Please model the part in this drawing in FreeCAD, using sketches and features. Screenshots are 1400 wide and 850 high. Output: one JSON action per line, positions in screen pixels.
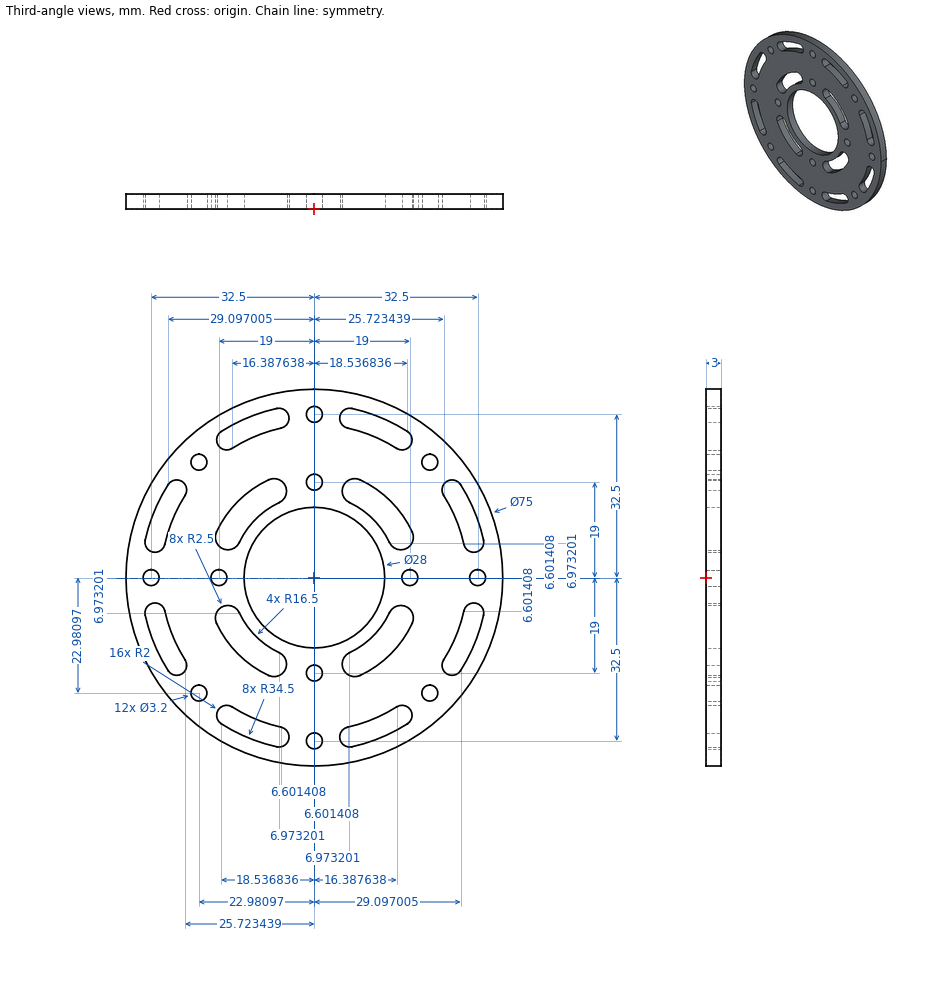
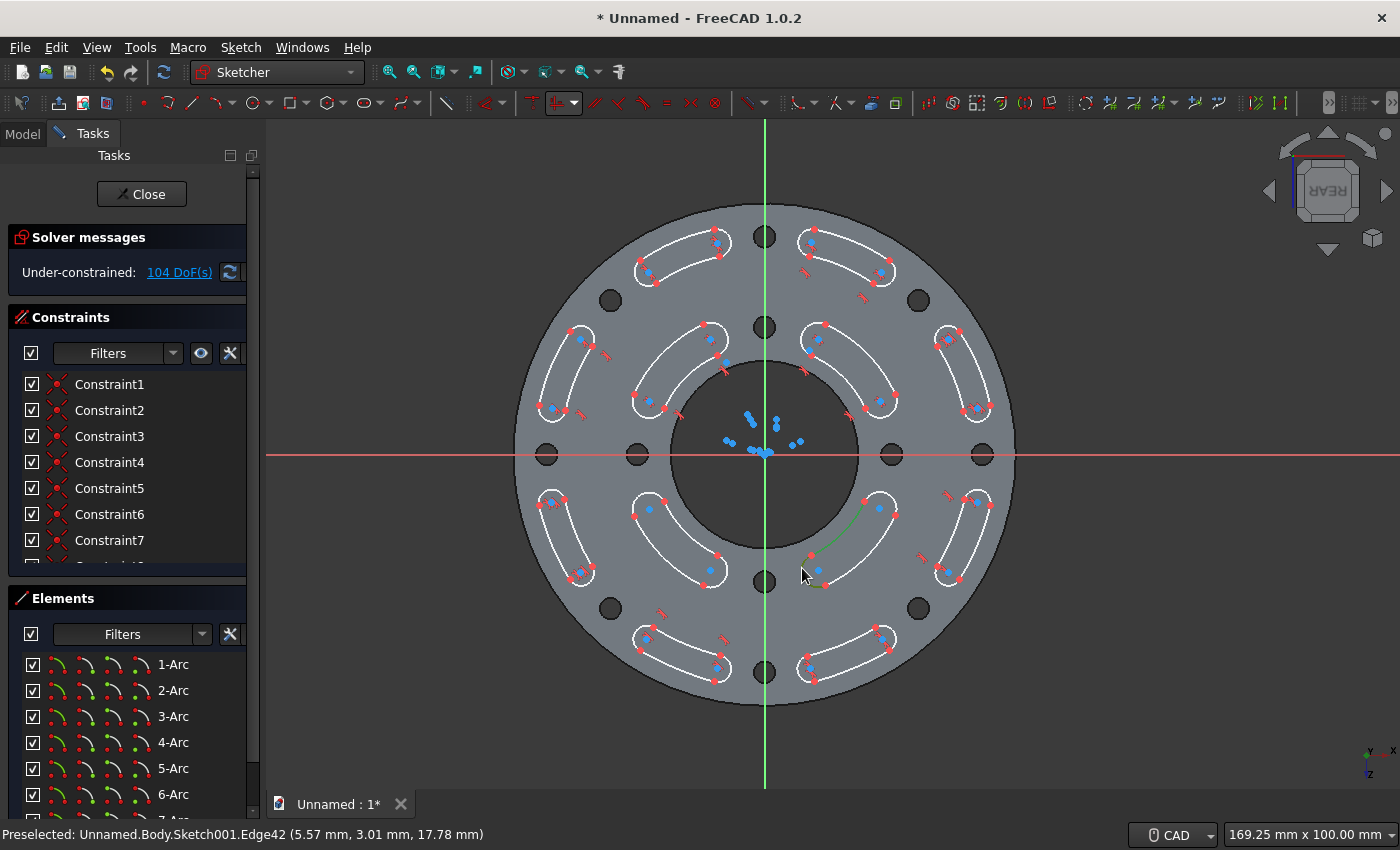
{"action": "left_click", "coordinate": [644, 104]}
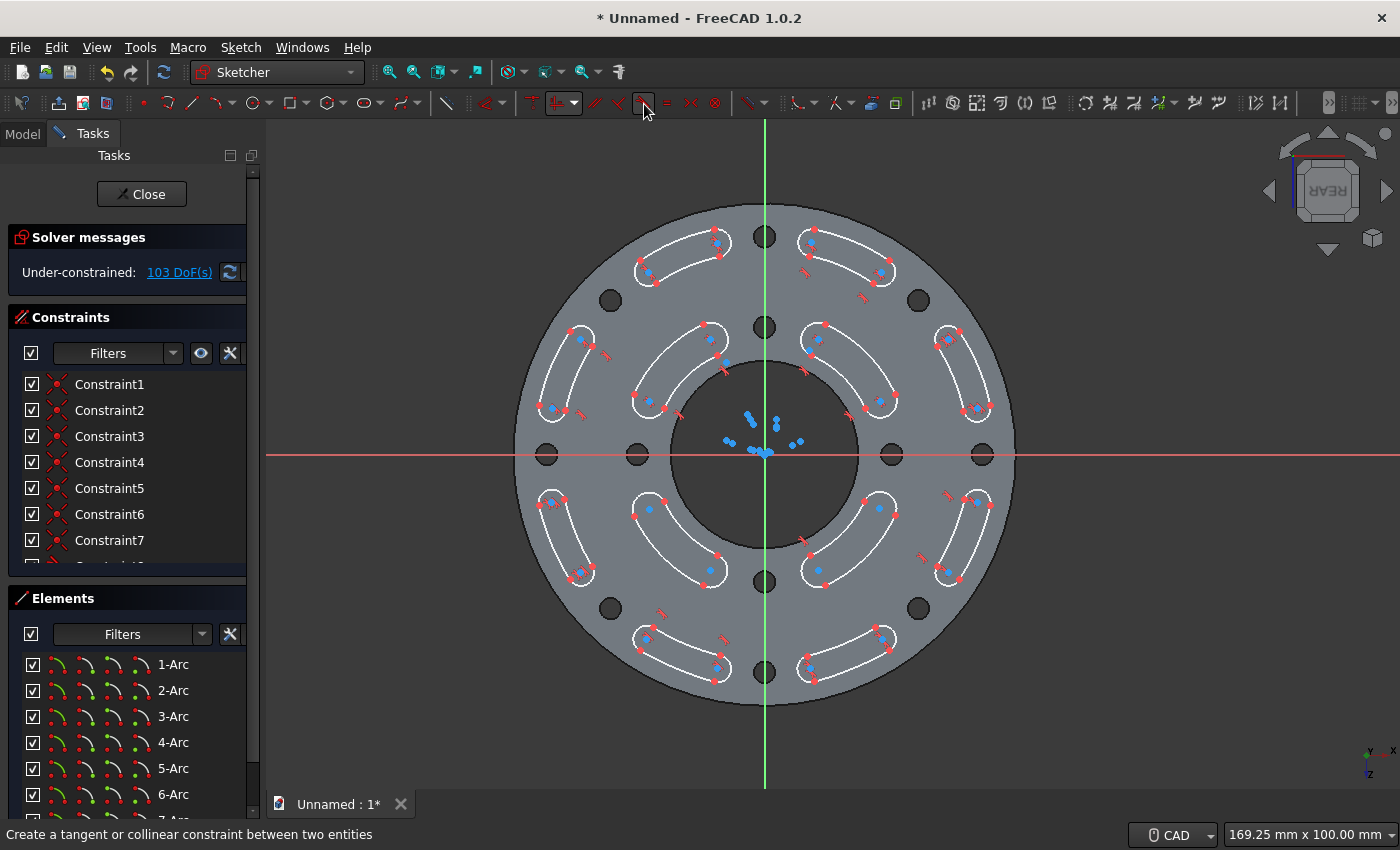
{"action": "left_click", "coordinate": [831, 543]}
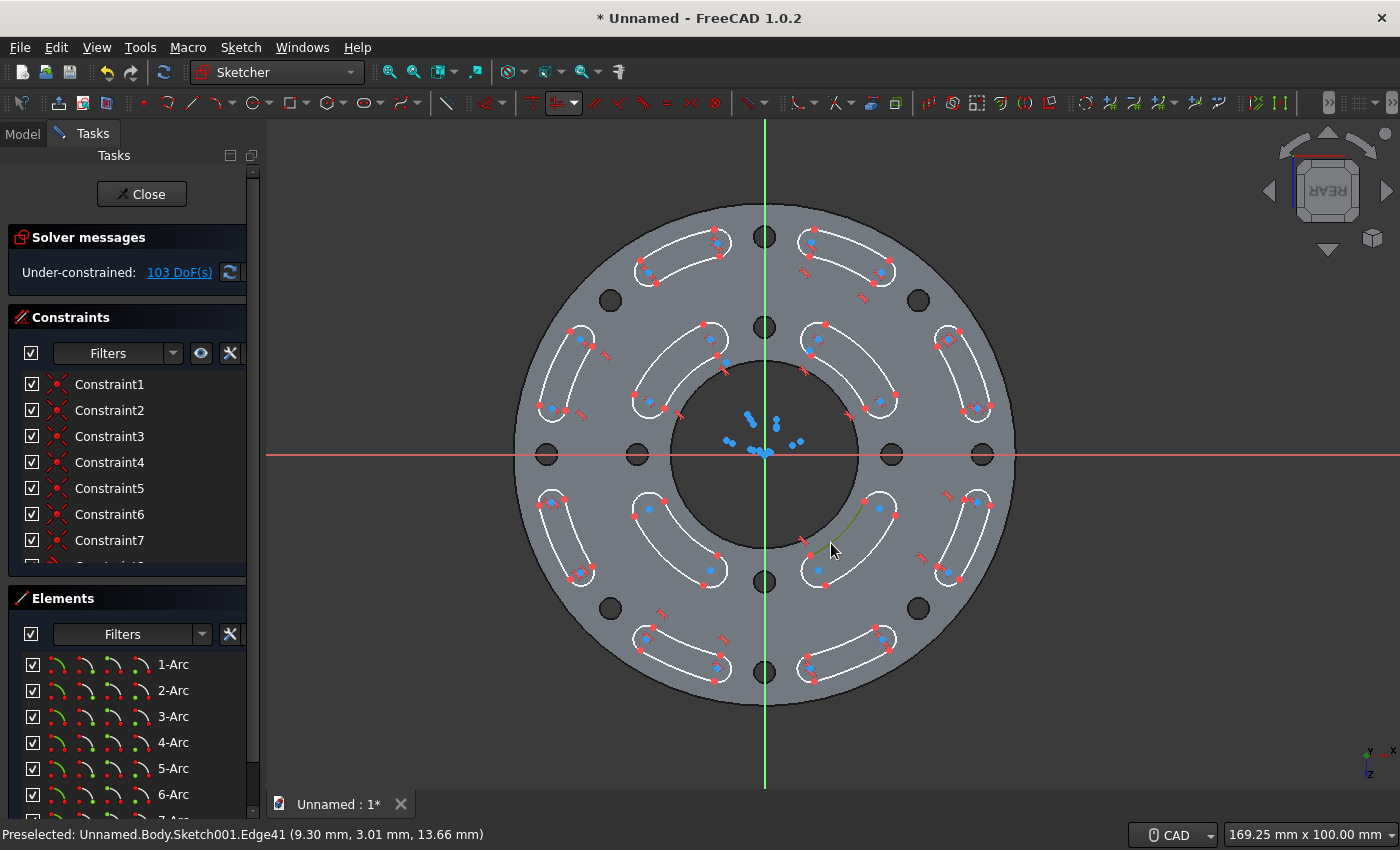
{"action": "left_click", "coordinate": [894, 501]}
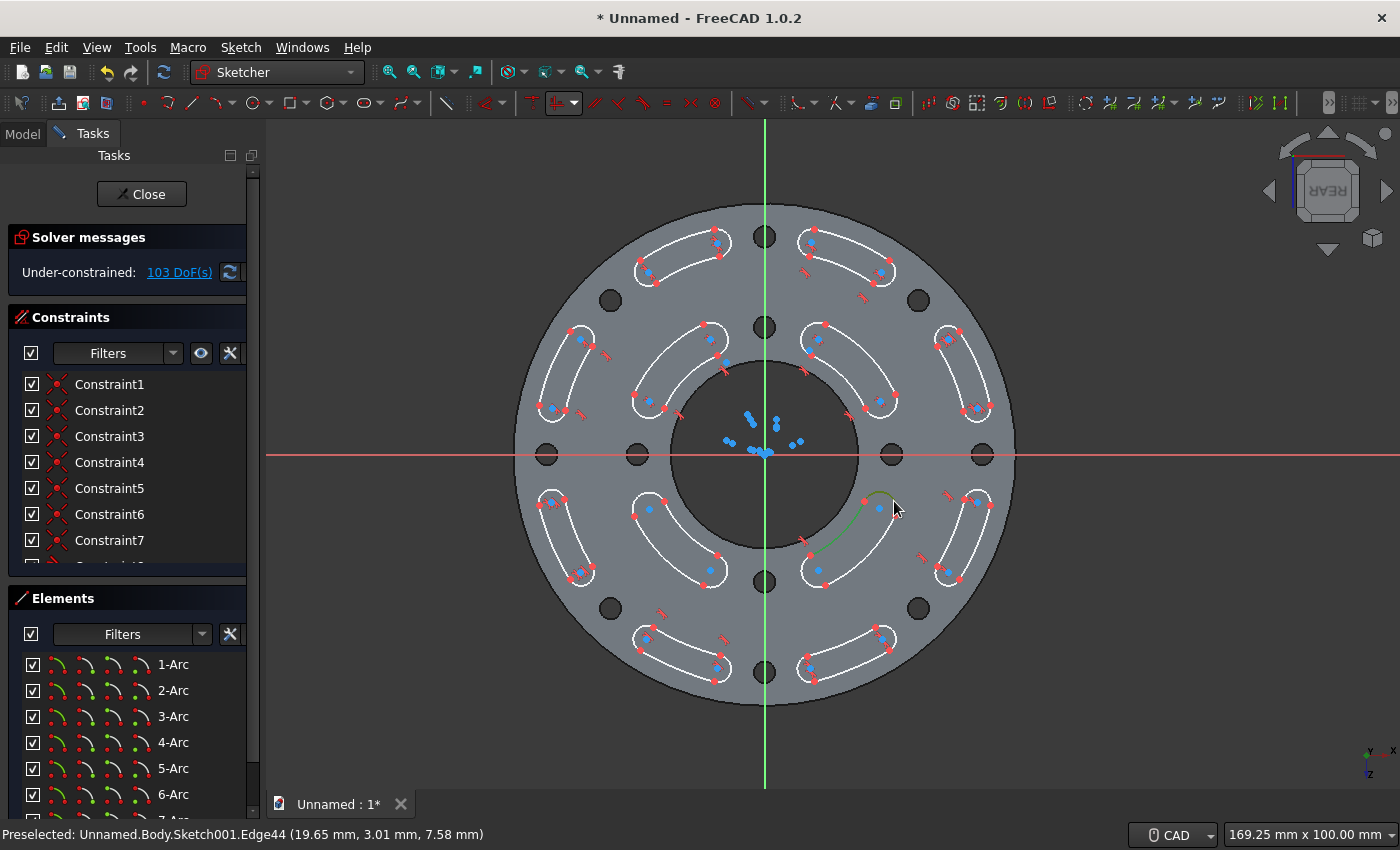
{"action": "left_click", "coordinate": [644, 104]}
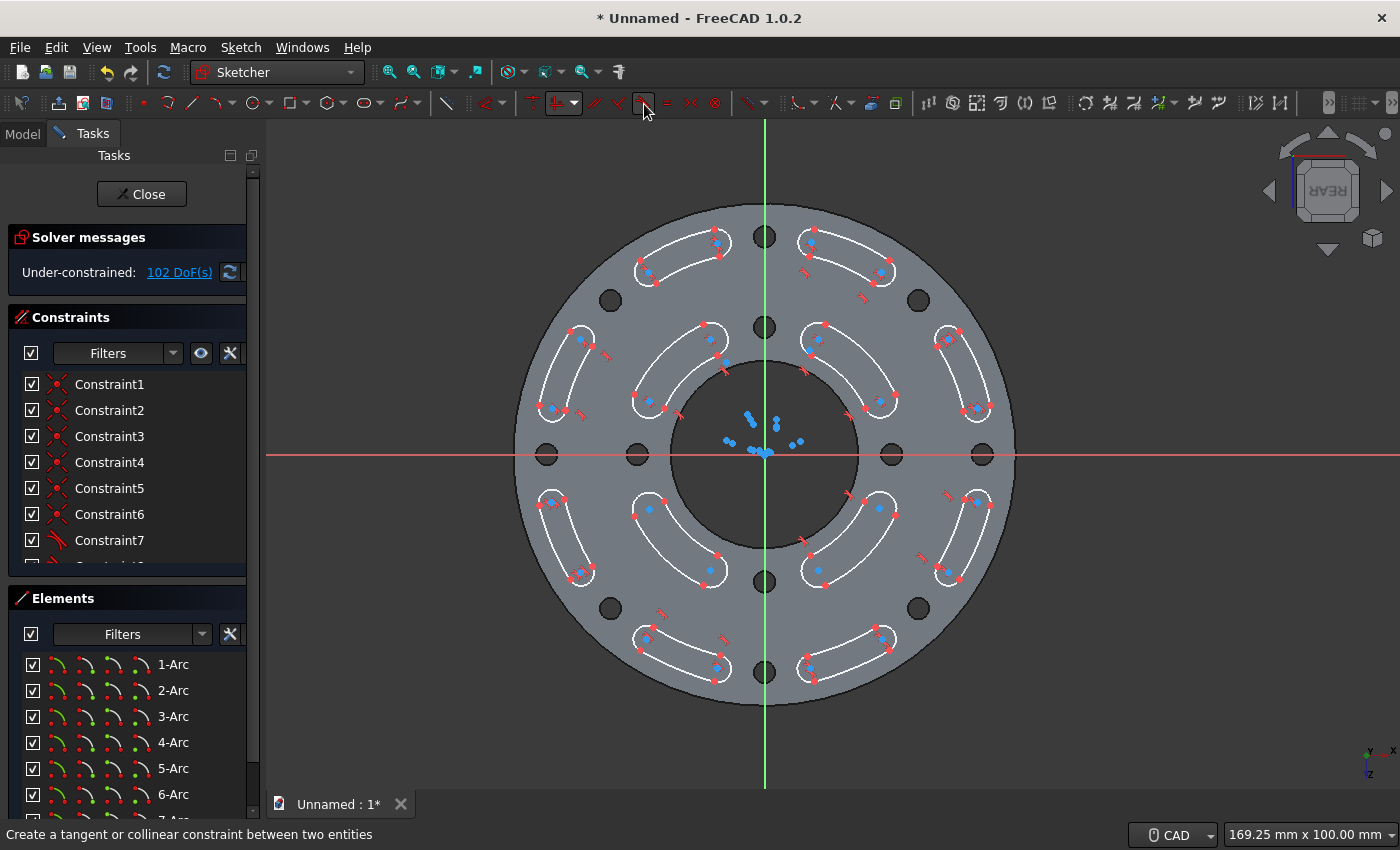
{"action": "left_click", "coordinate": [802, 568]}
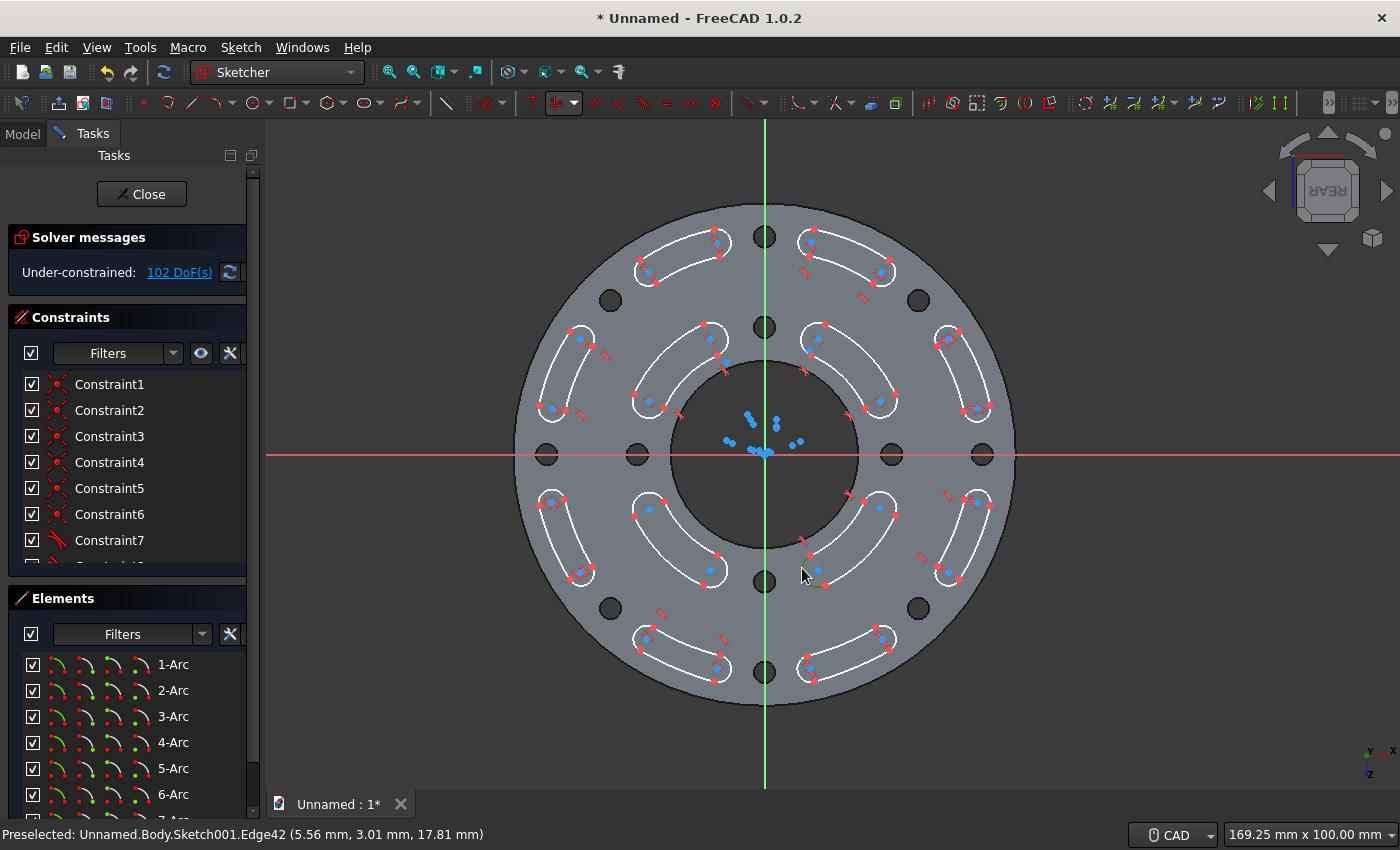
{"action": "left_click", "coordinate": [851, 570]}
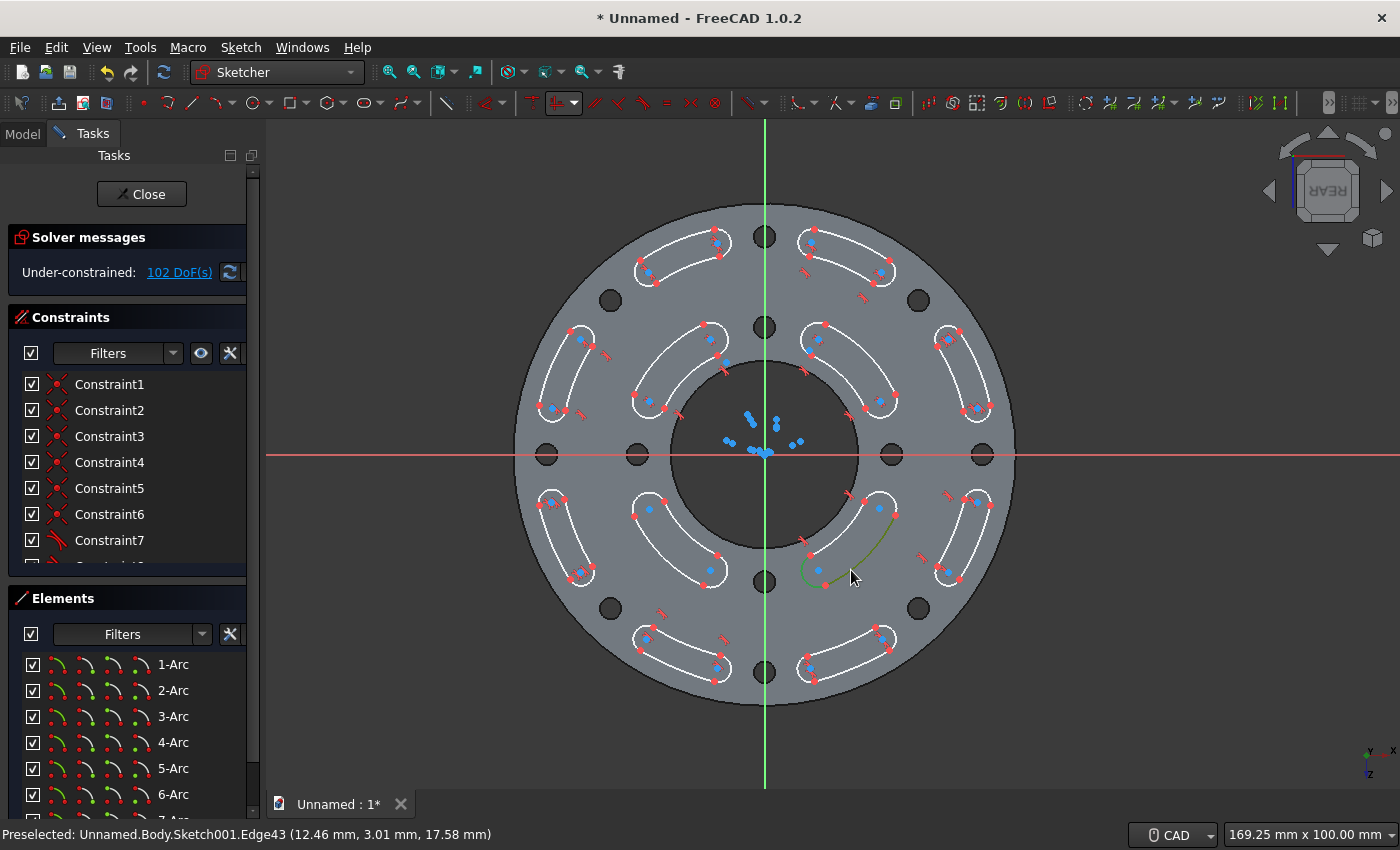
{"action": "left_click", "coordinate": [644, 104]}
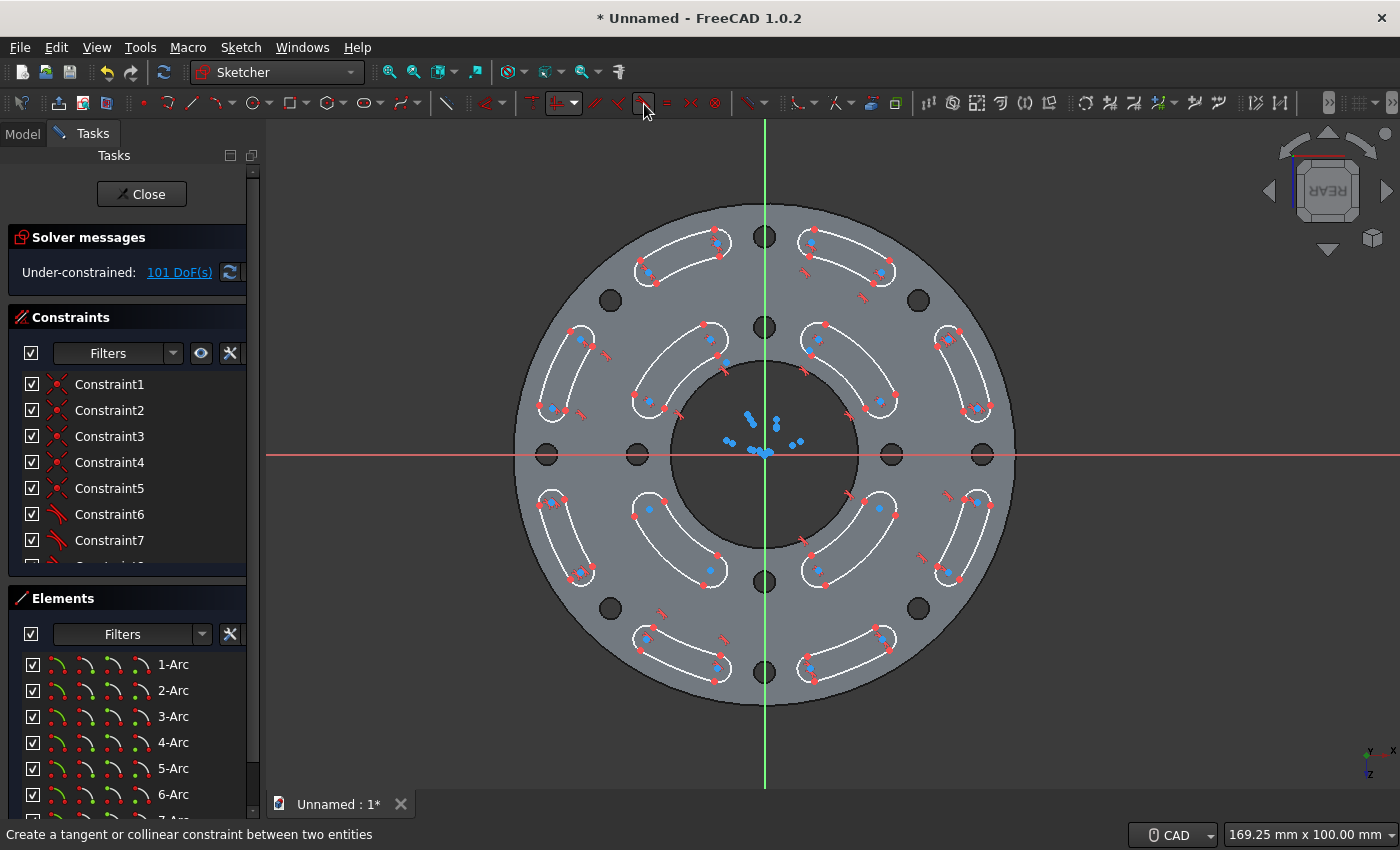
{"action": "left_click", "coordinate": [851, 570]}